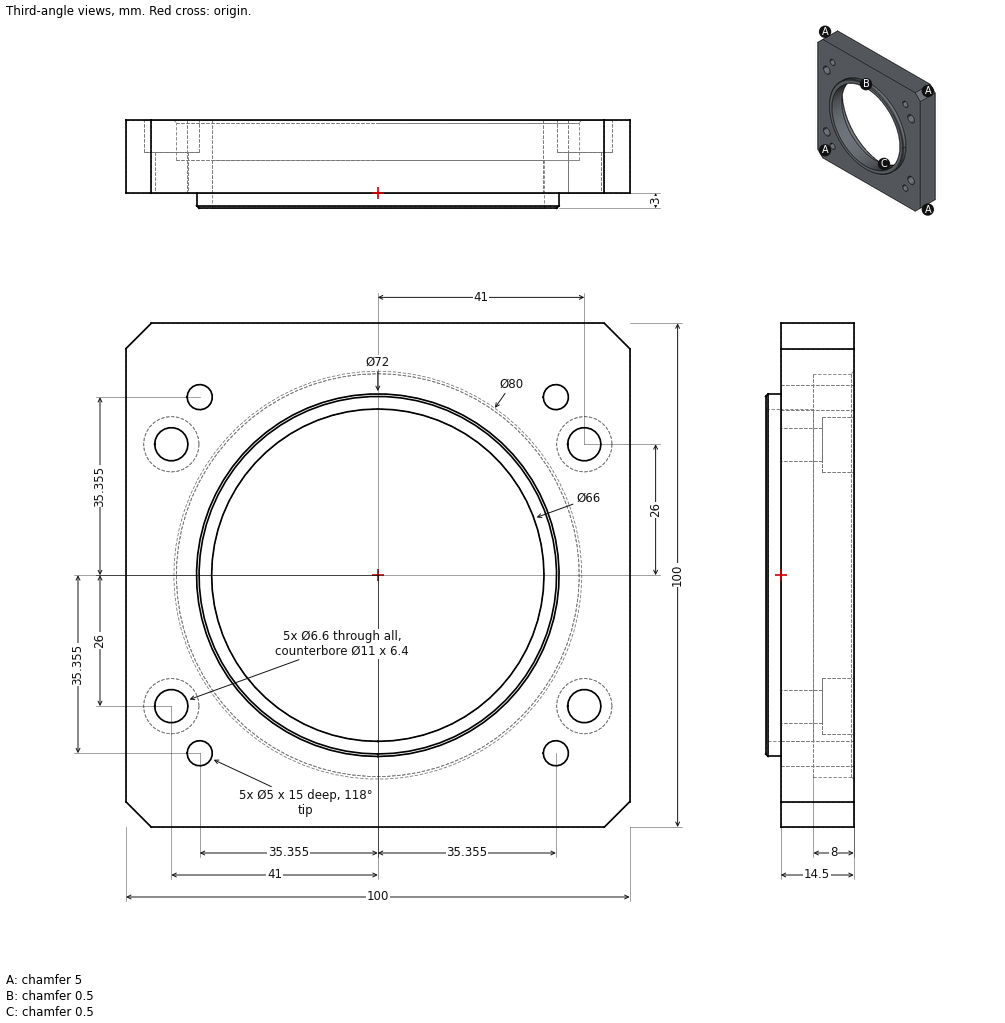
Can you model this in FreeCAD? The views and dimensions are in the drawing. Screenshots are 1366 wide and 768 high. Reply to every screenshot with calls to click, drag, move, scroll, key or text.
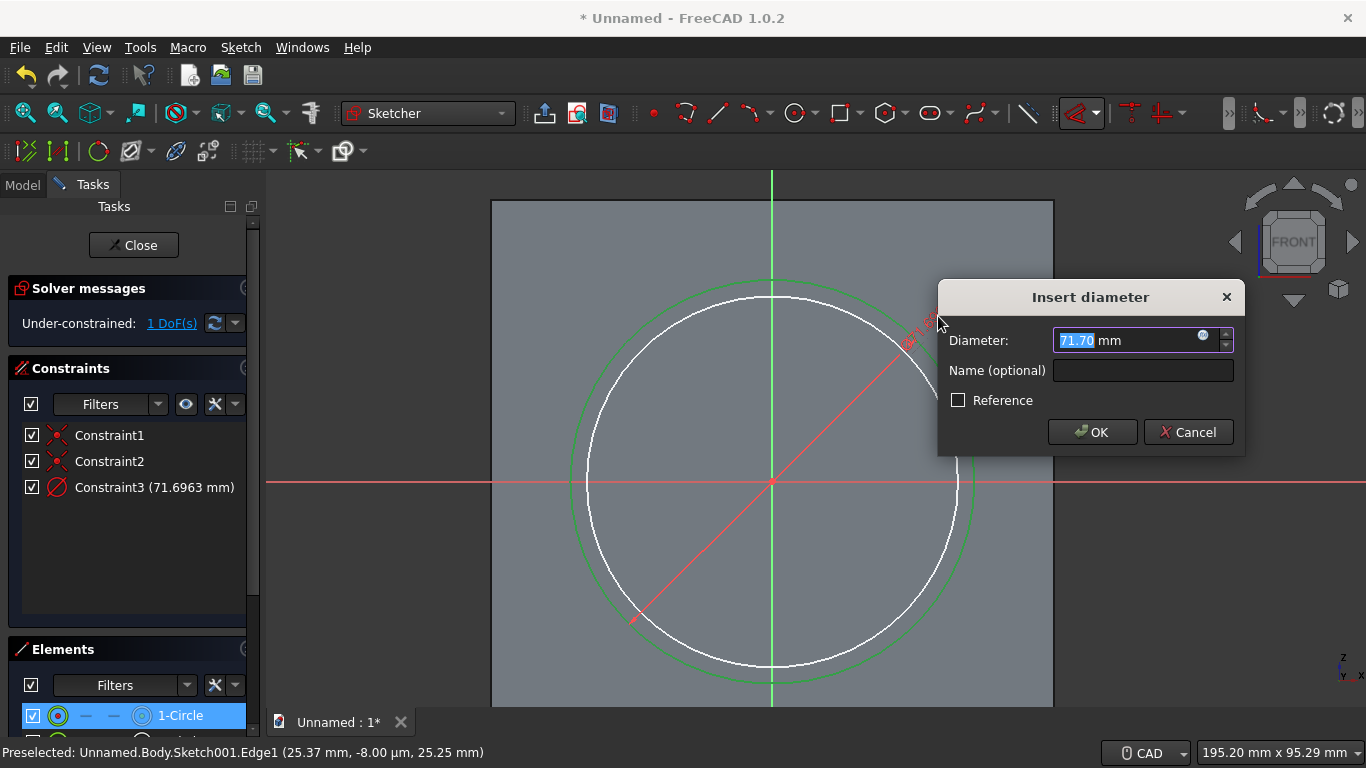
text(72)
key(Return)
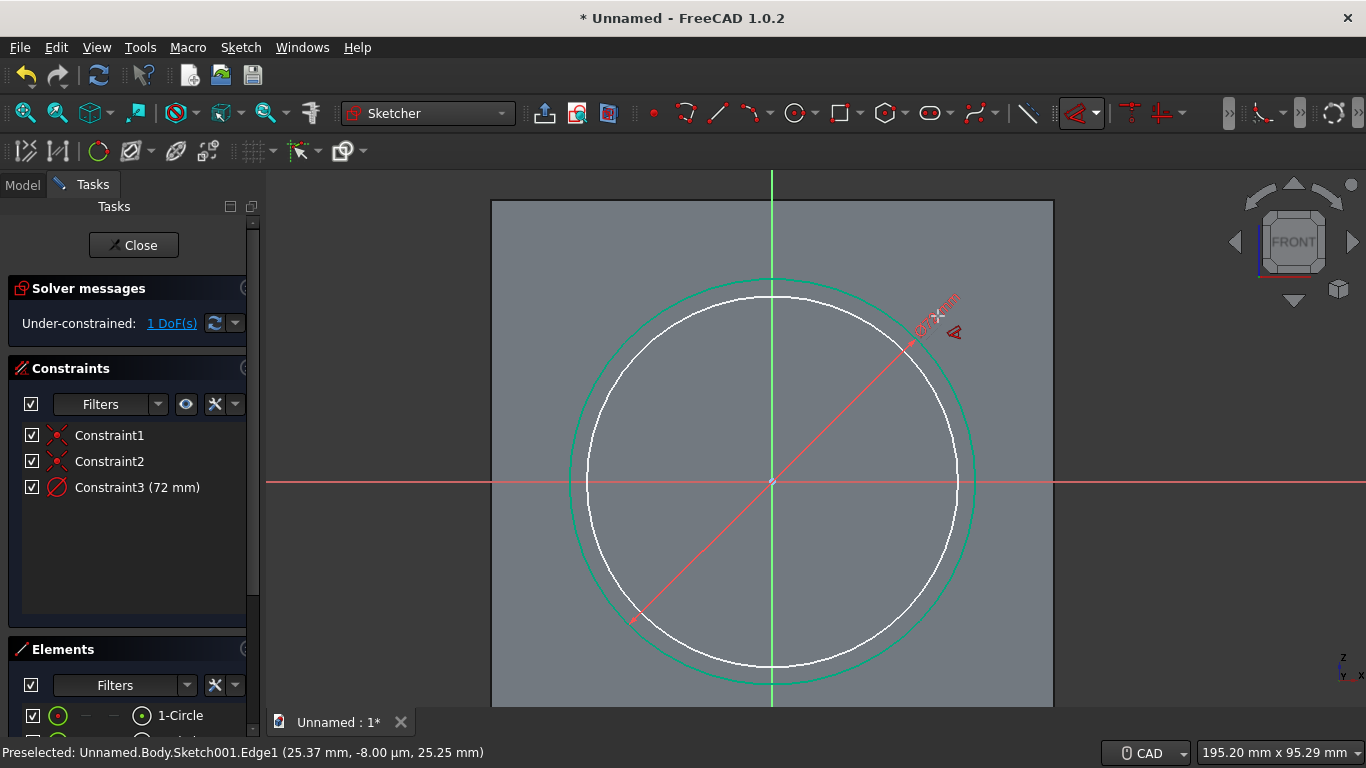
click(903, 350)
click(981, 420)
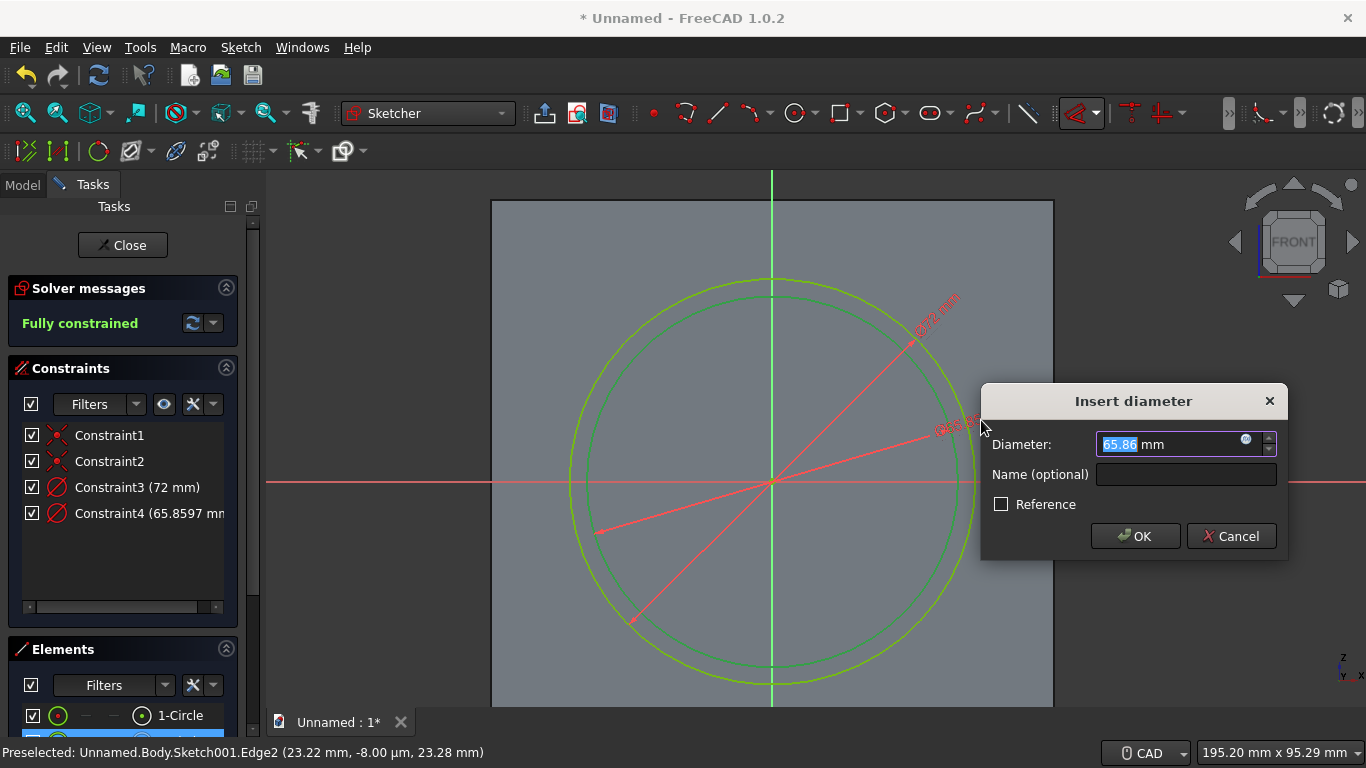
text(66)
key(Return)
key(Escape)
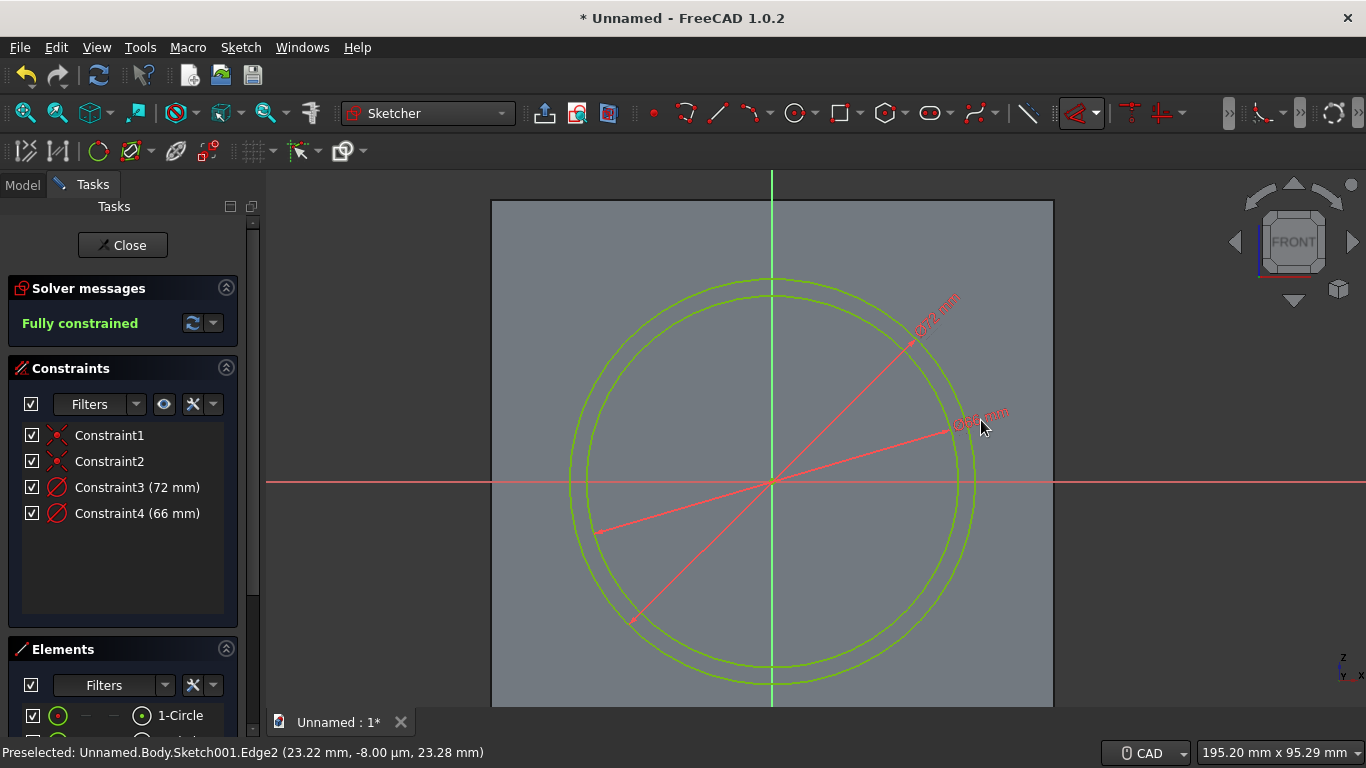
click(123, 245)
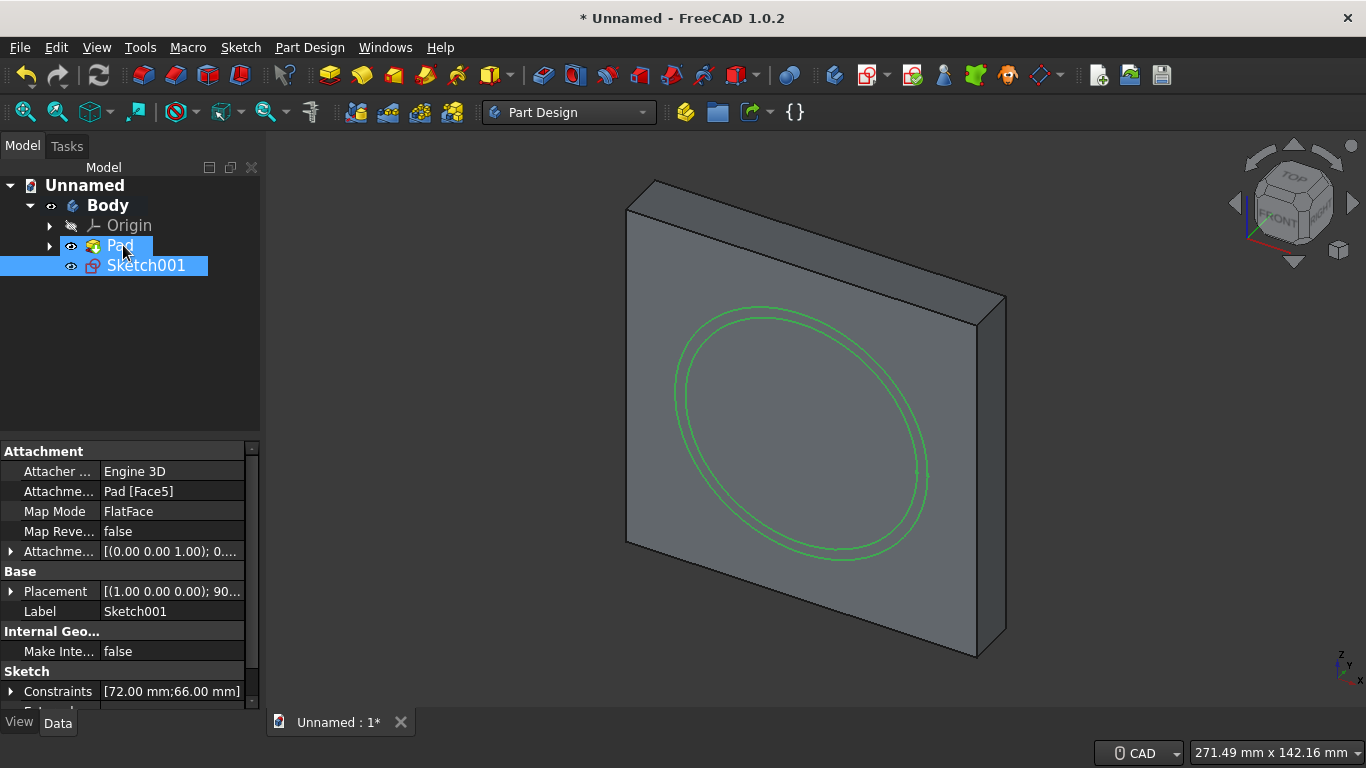
click(330, 76)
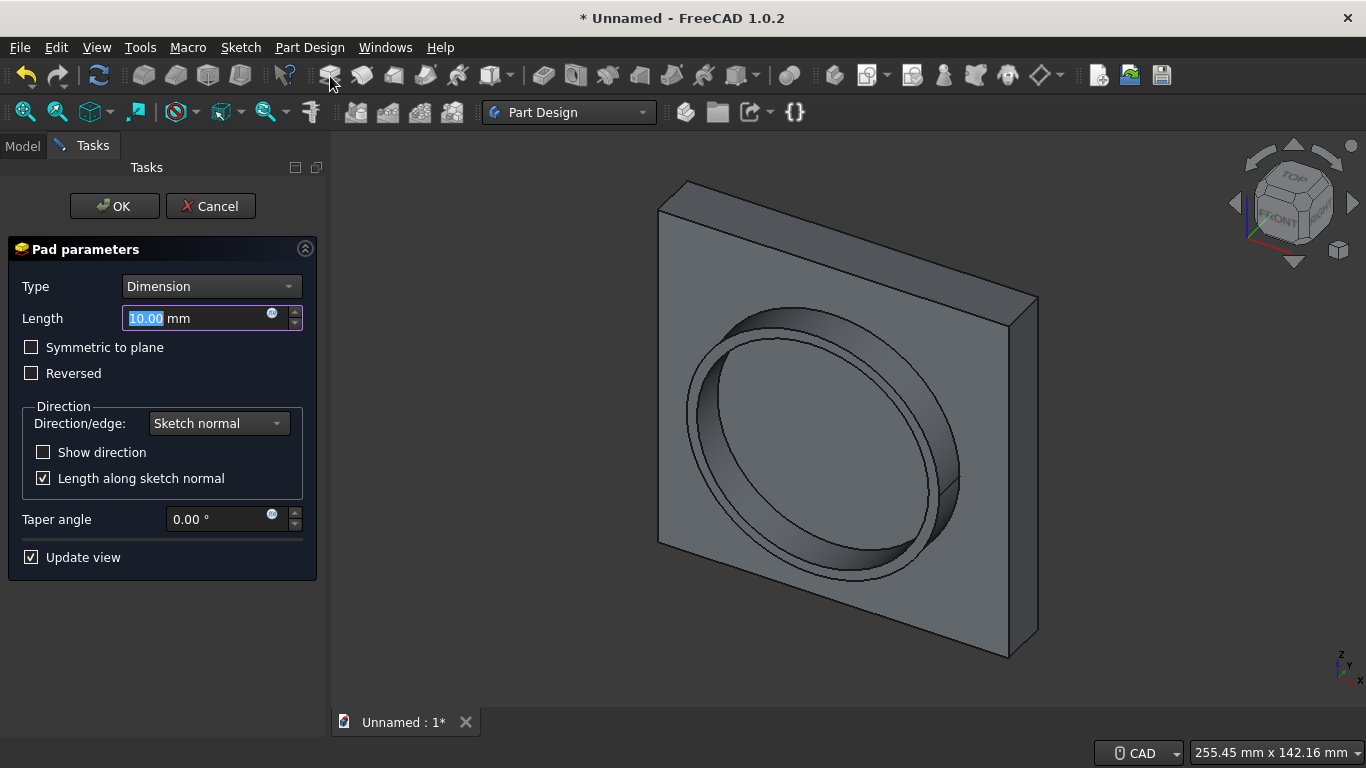
text(3)
key(Tab)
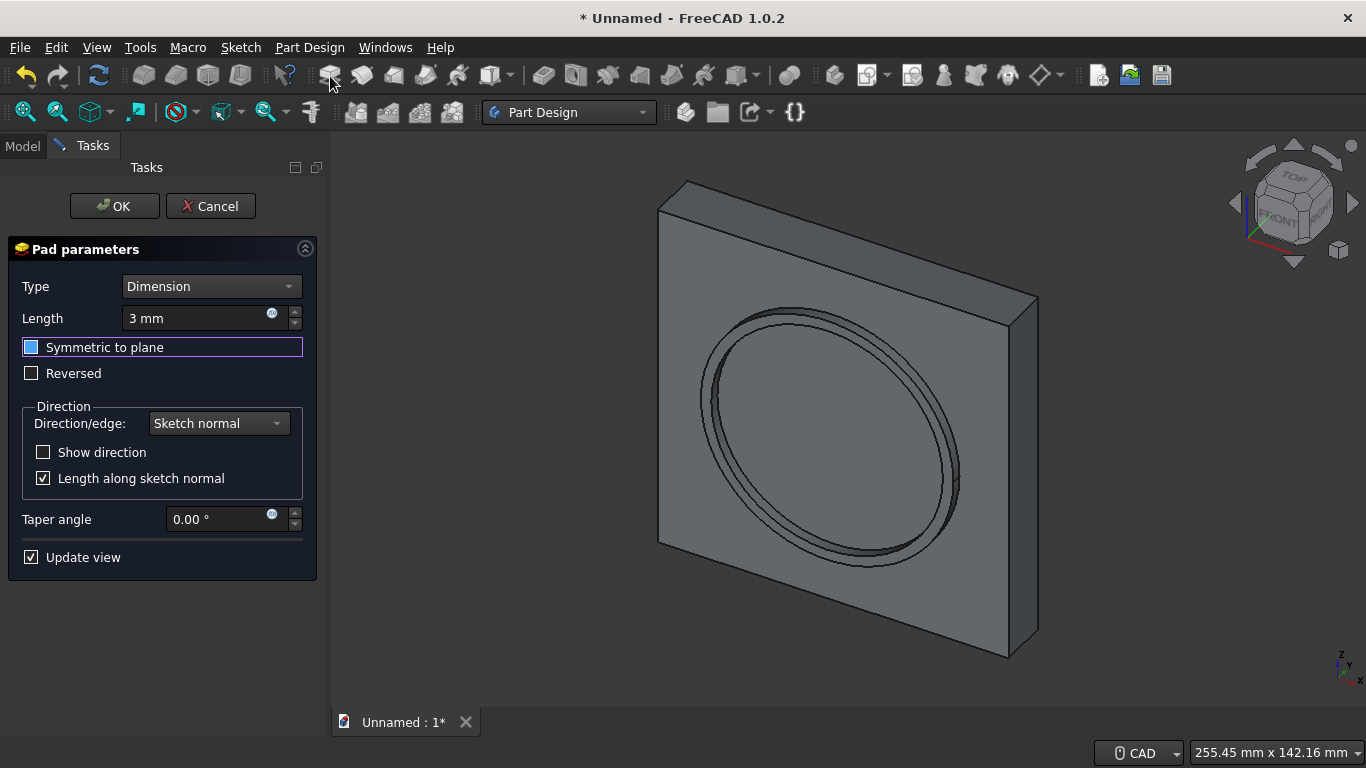
click(115, 206)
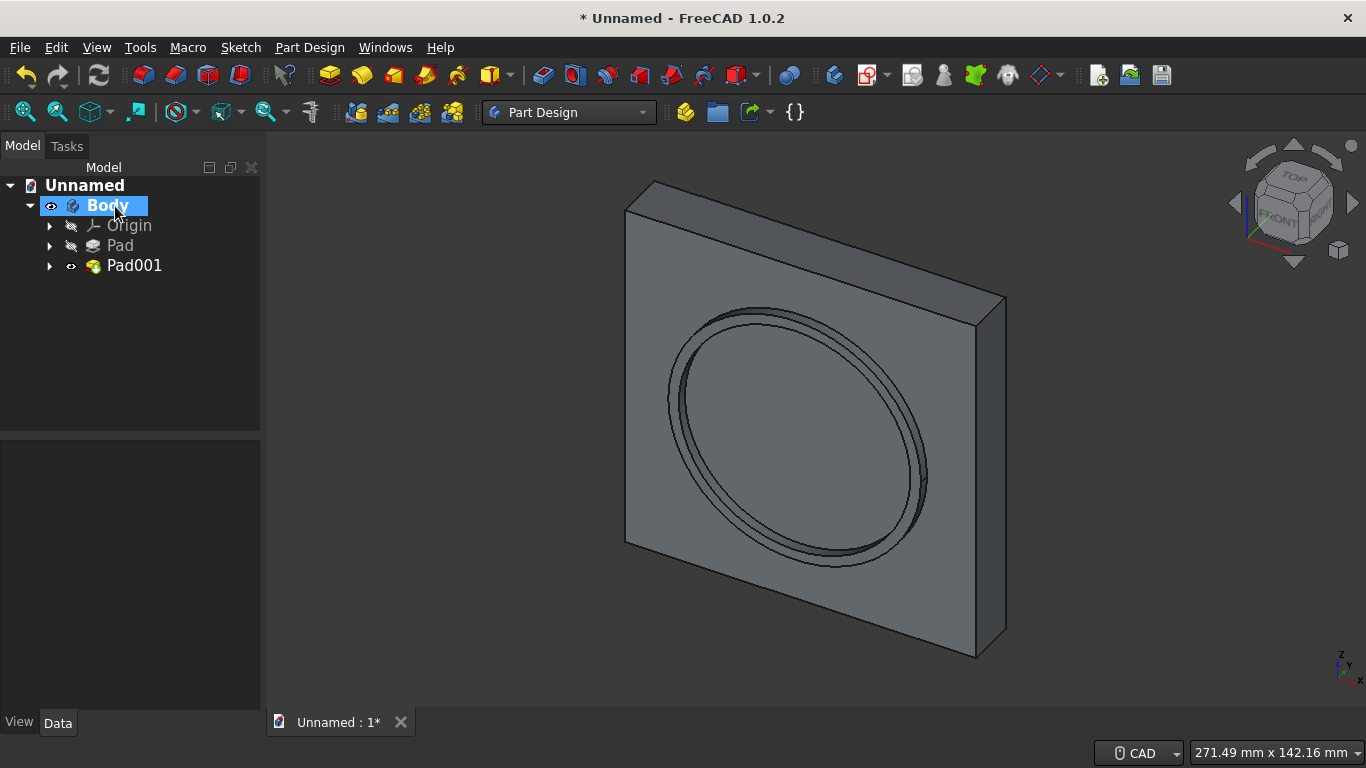
click(901, 609)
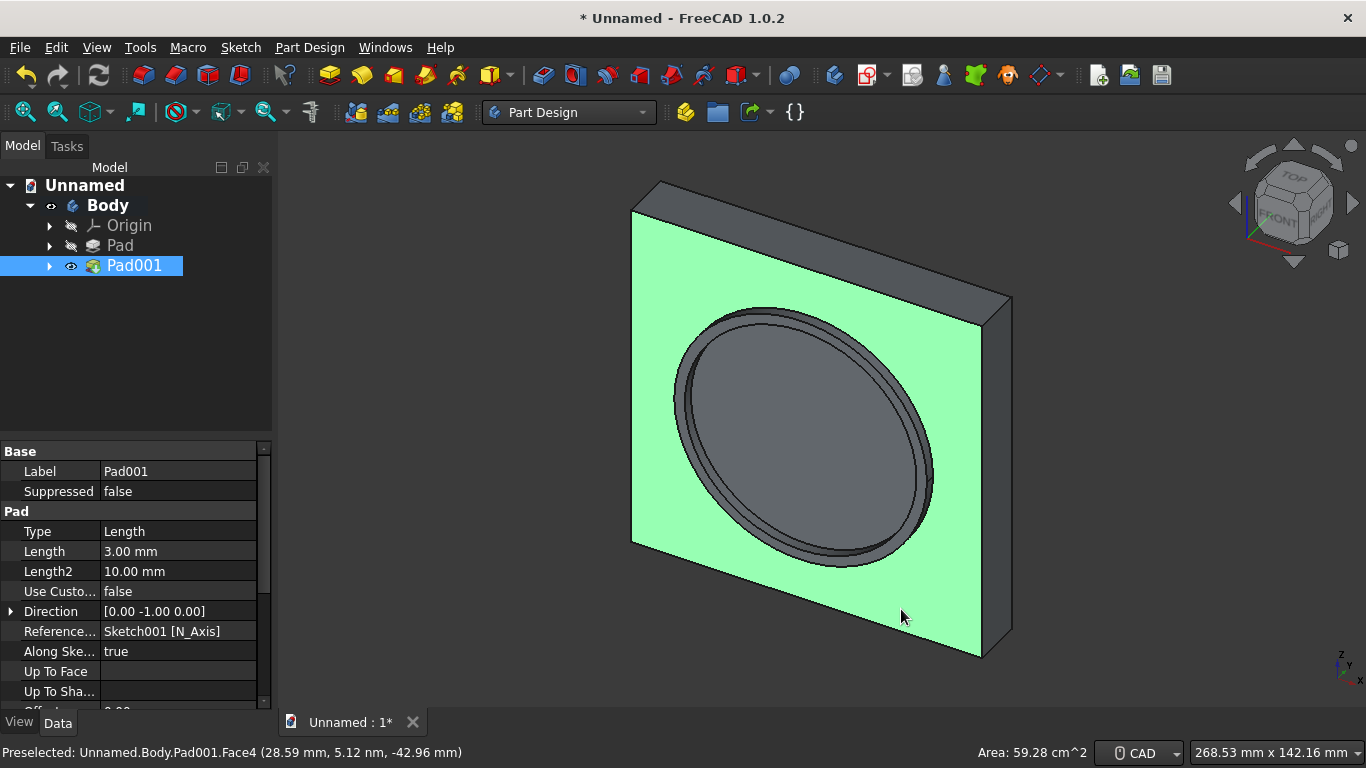
click(868, 76)